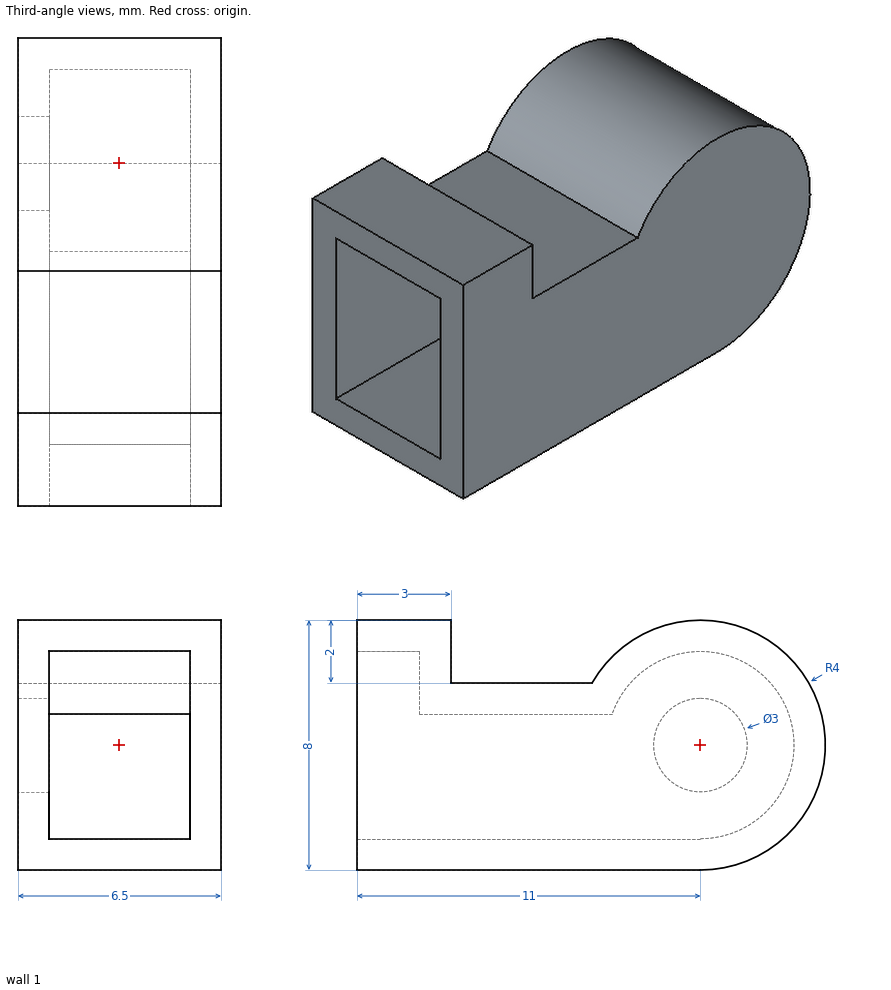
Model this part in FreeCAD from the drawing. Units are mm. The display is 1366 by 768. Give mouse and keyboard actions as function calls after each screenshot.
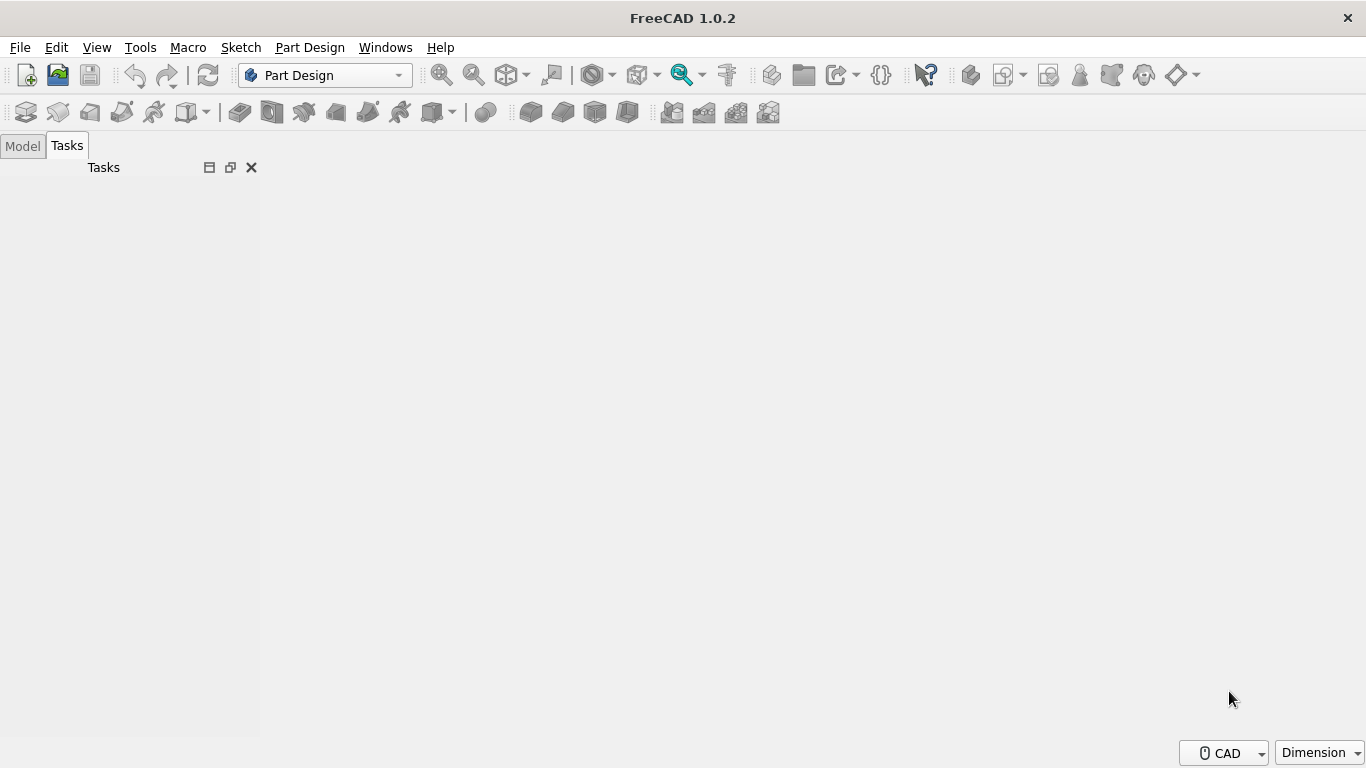
click(26, 76)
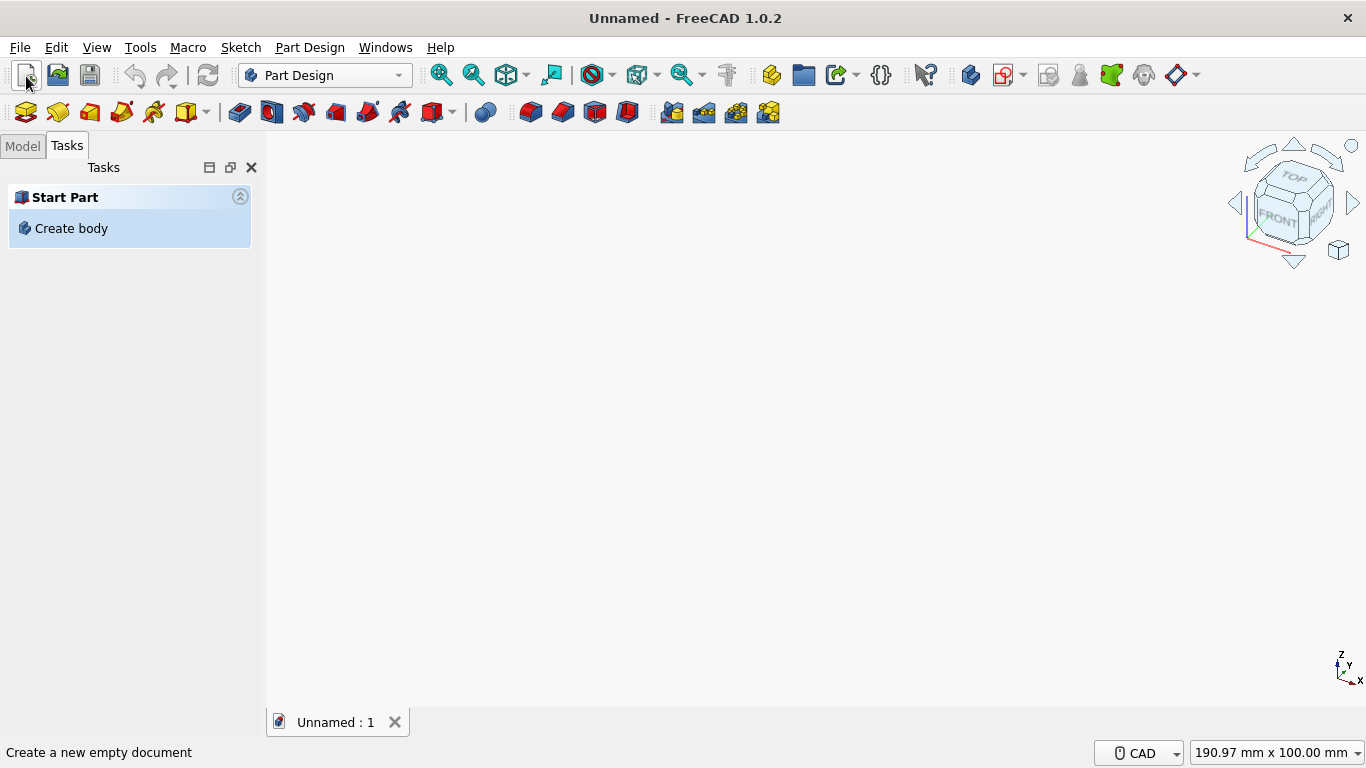
click(1004, 76)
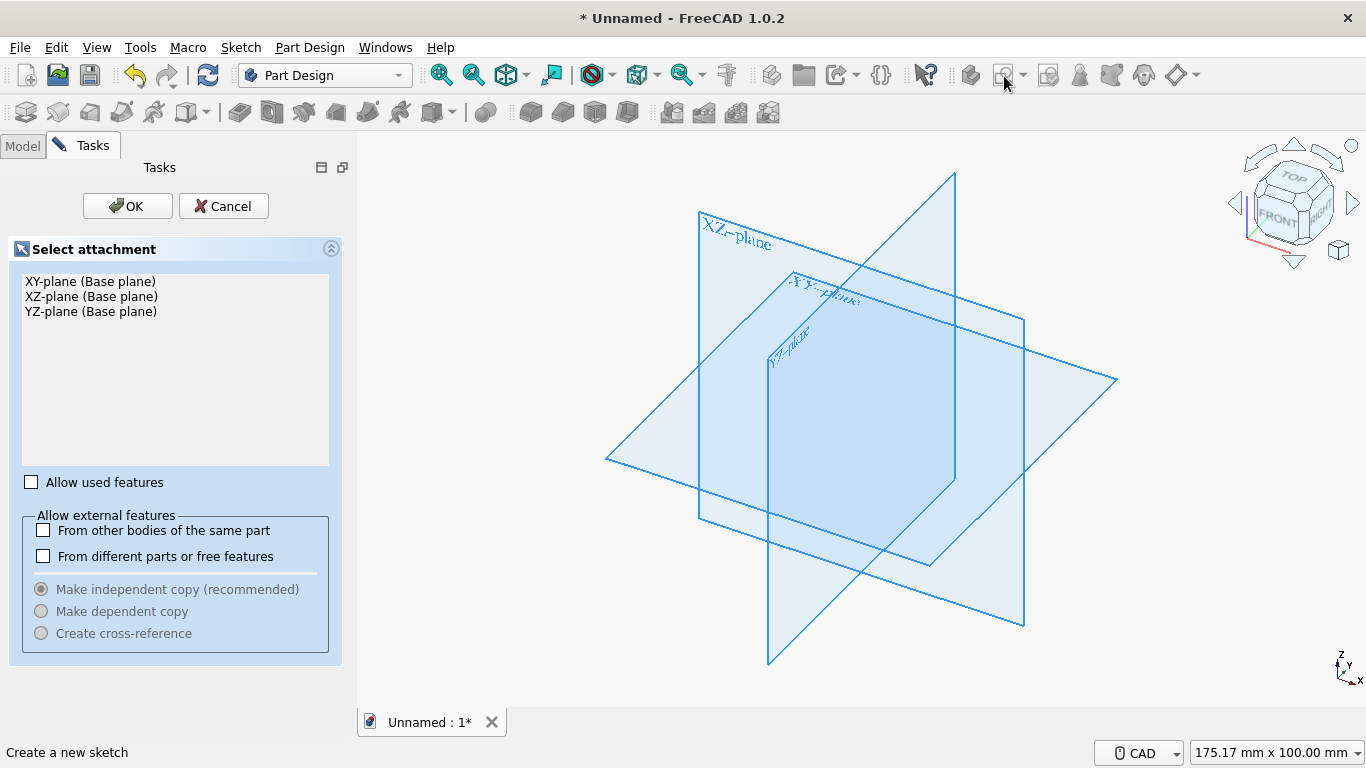
click(82, 312)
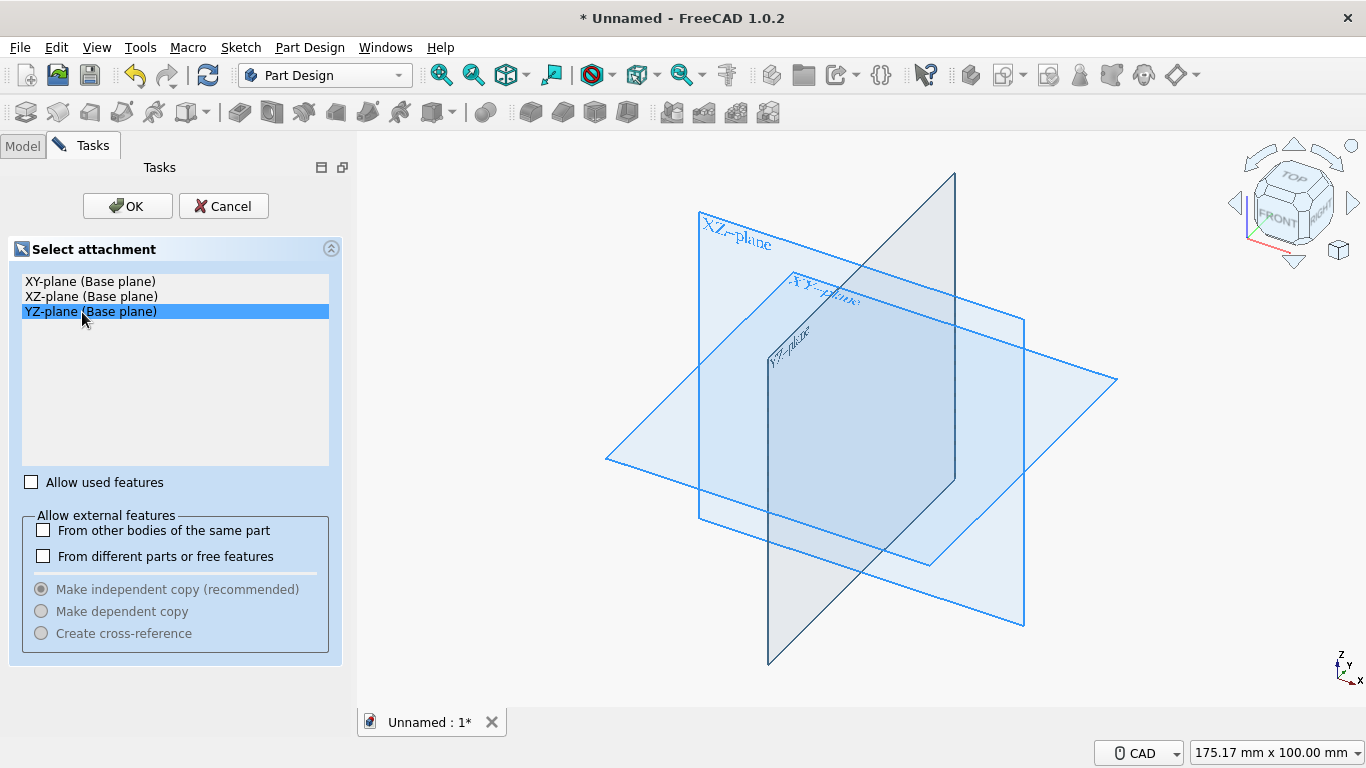
click(128, 206)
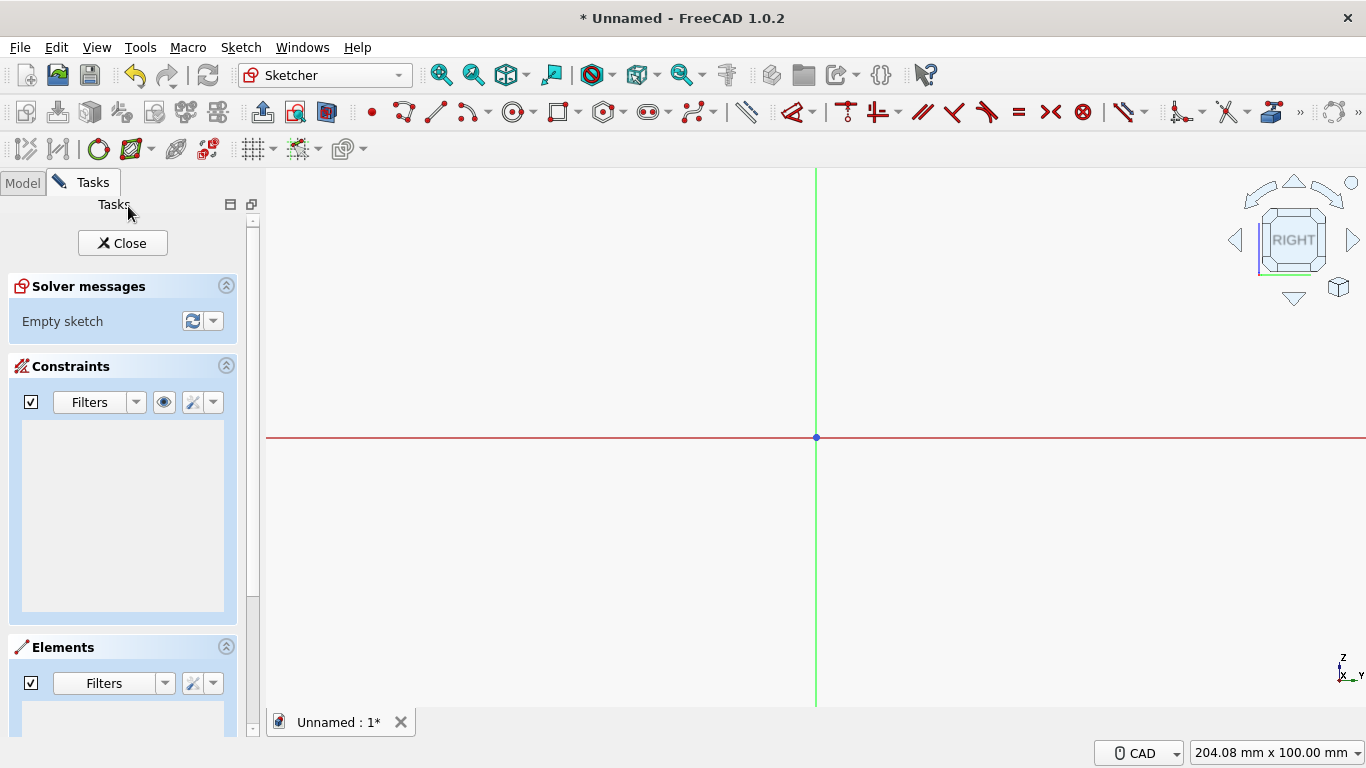
scroll(803, 437, up, 10)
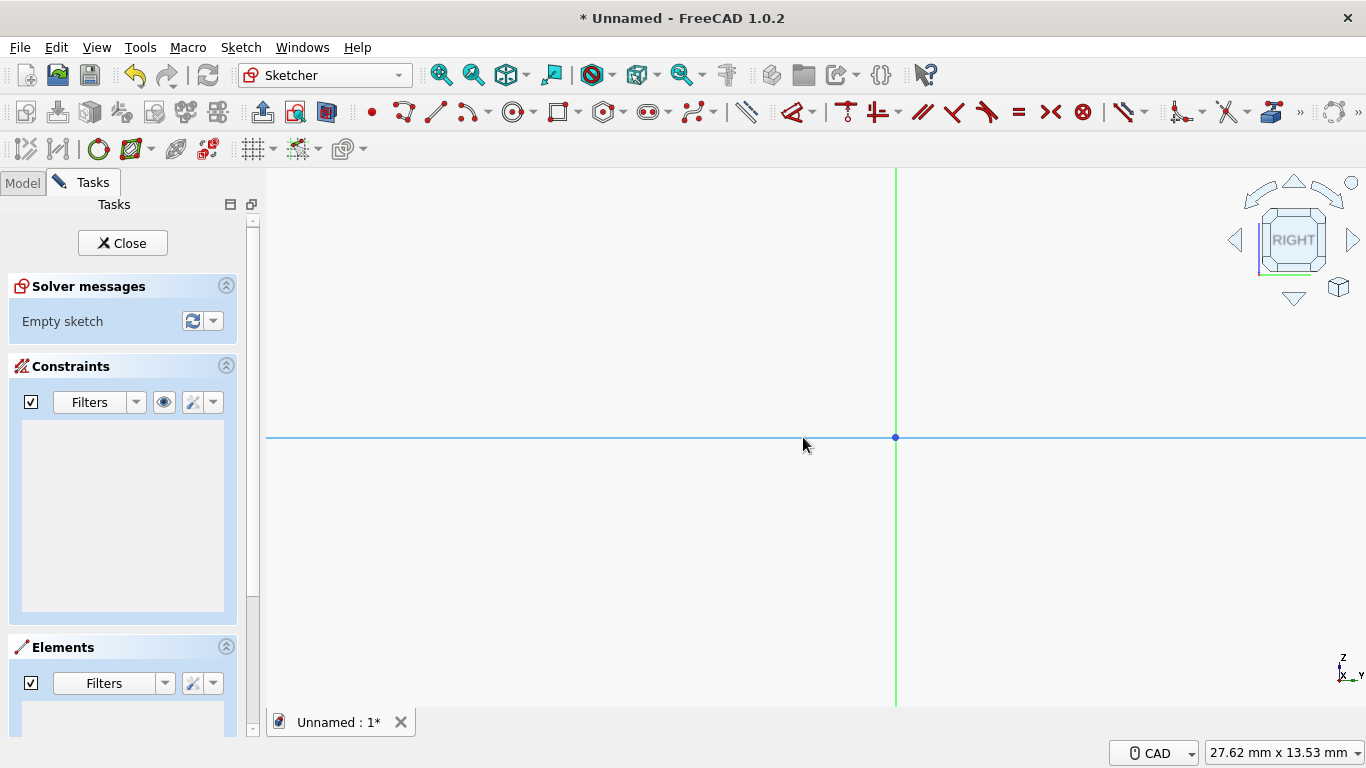
key(g)
key(m)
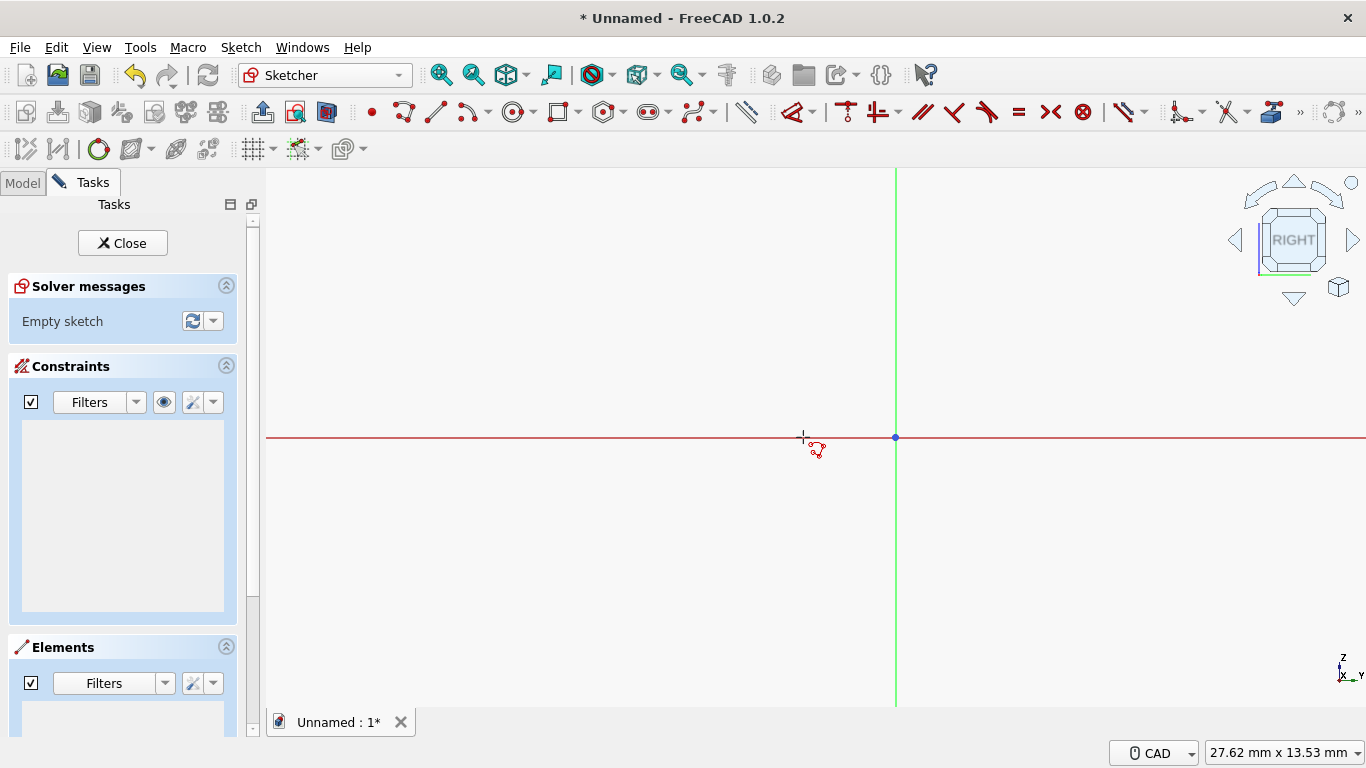
click(758, 358)
click(577, 358)
click(577, 278)
click(458, 278)
click(458, 597)
click(896, 597)
right_click(896, 597)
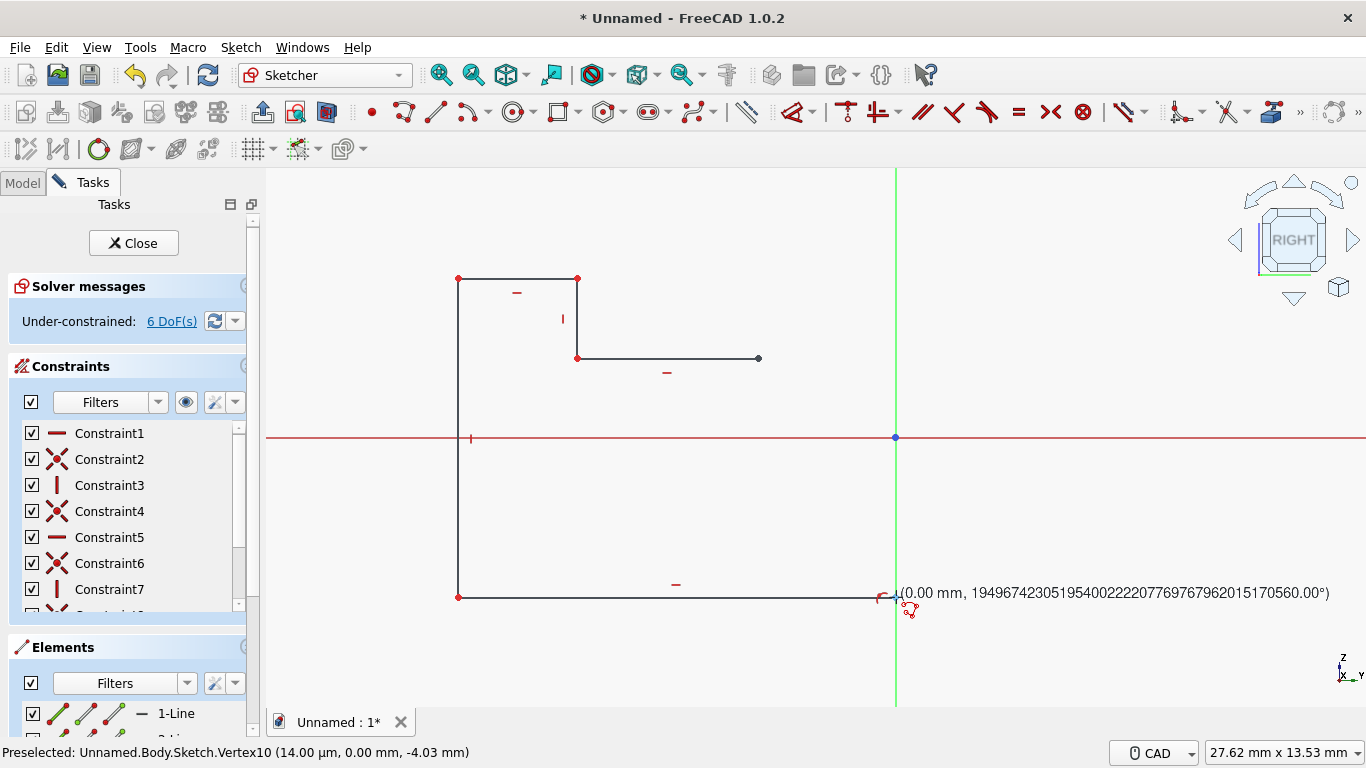
click(490, 112)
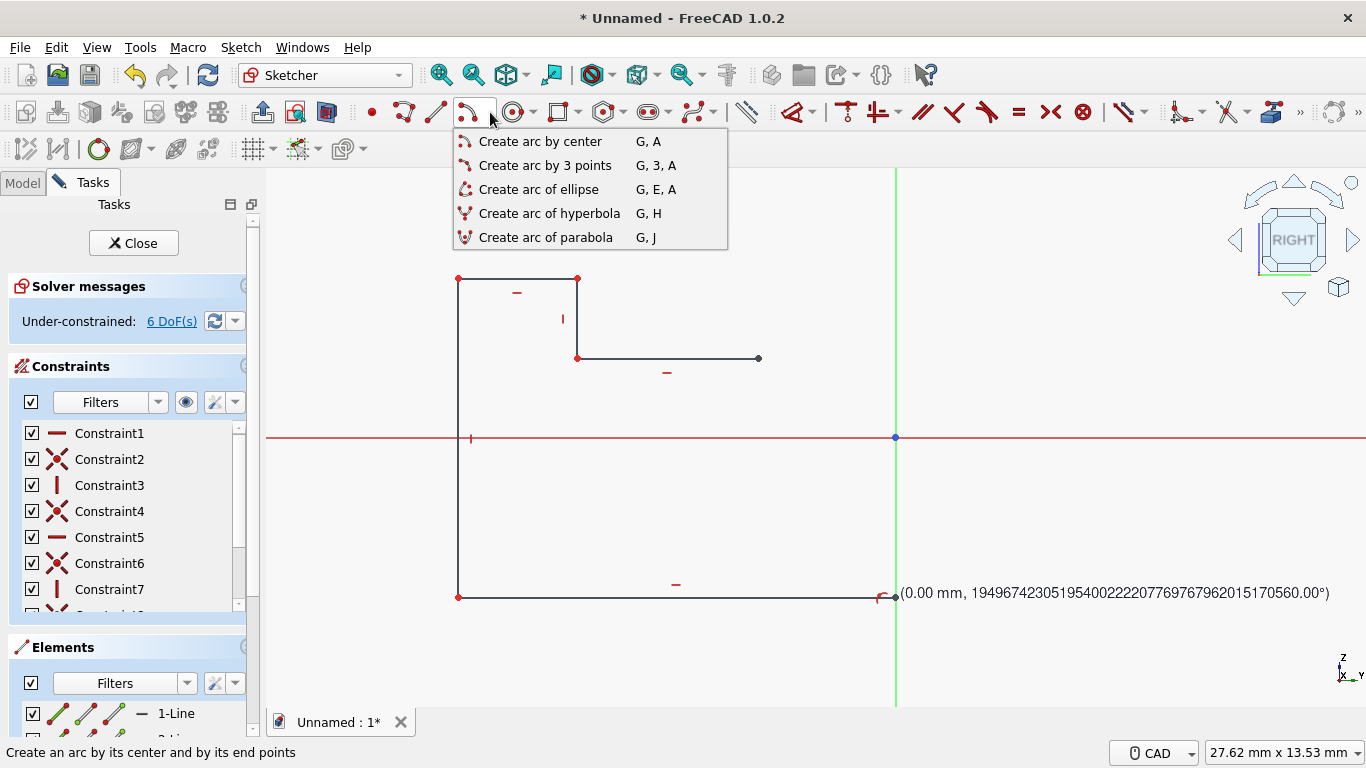
click(590, 165)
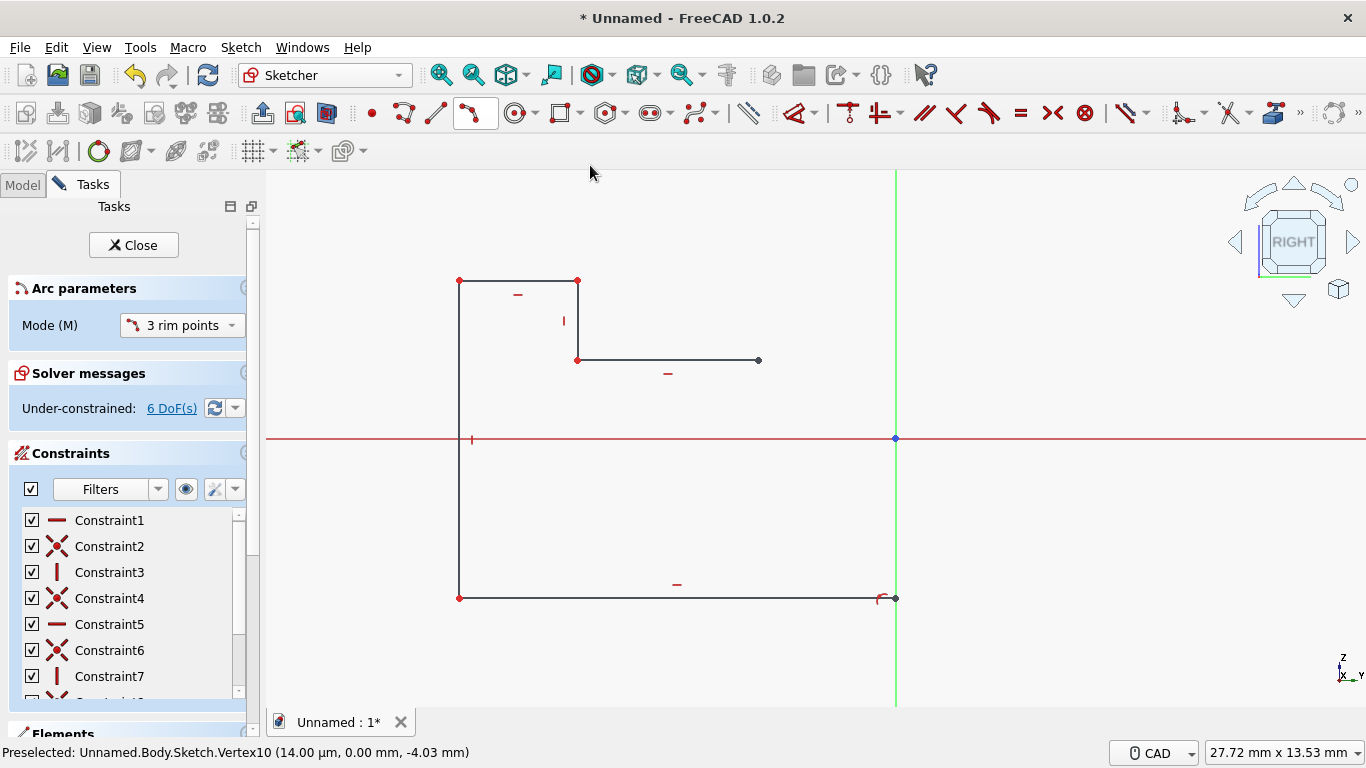
click(896, 598)
click(758, 360)
click(1033, 359)
key(Escape)